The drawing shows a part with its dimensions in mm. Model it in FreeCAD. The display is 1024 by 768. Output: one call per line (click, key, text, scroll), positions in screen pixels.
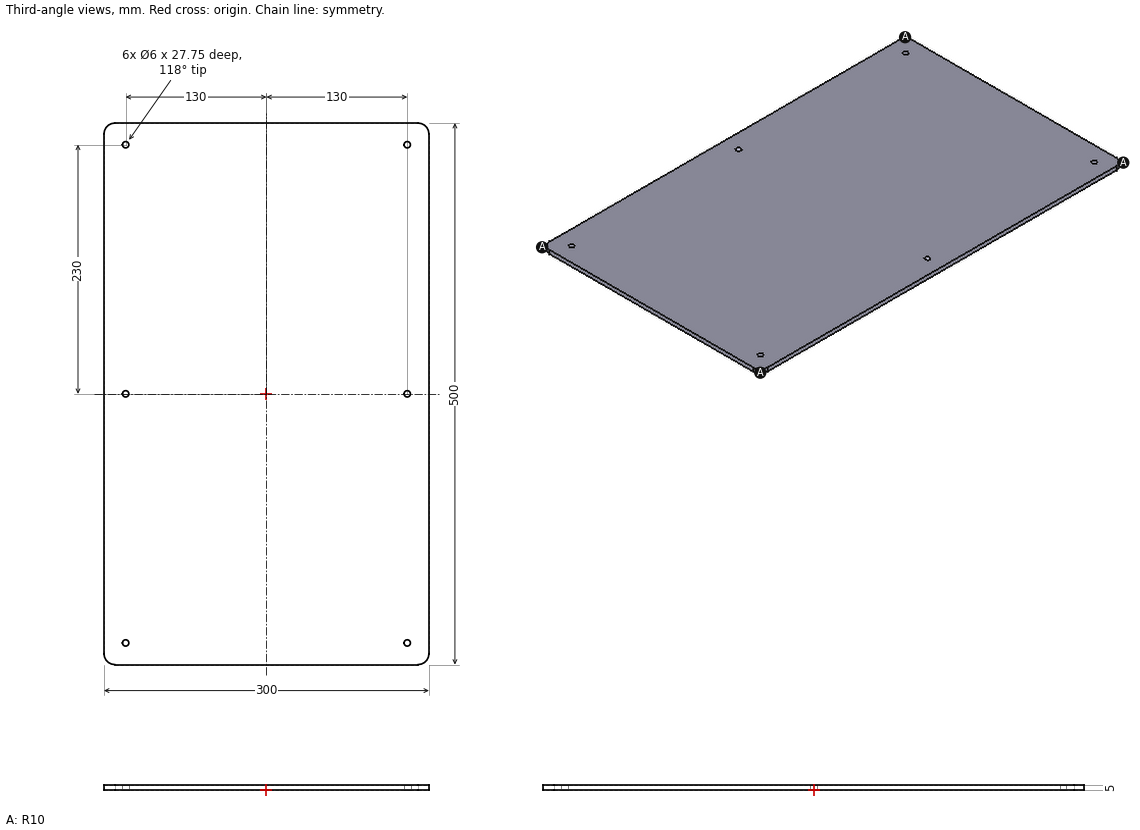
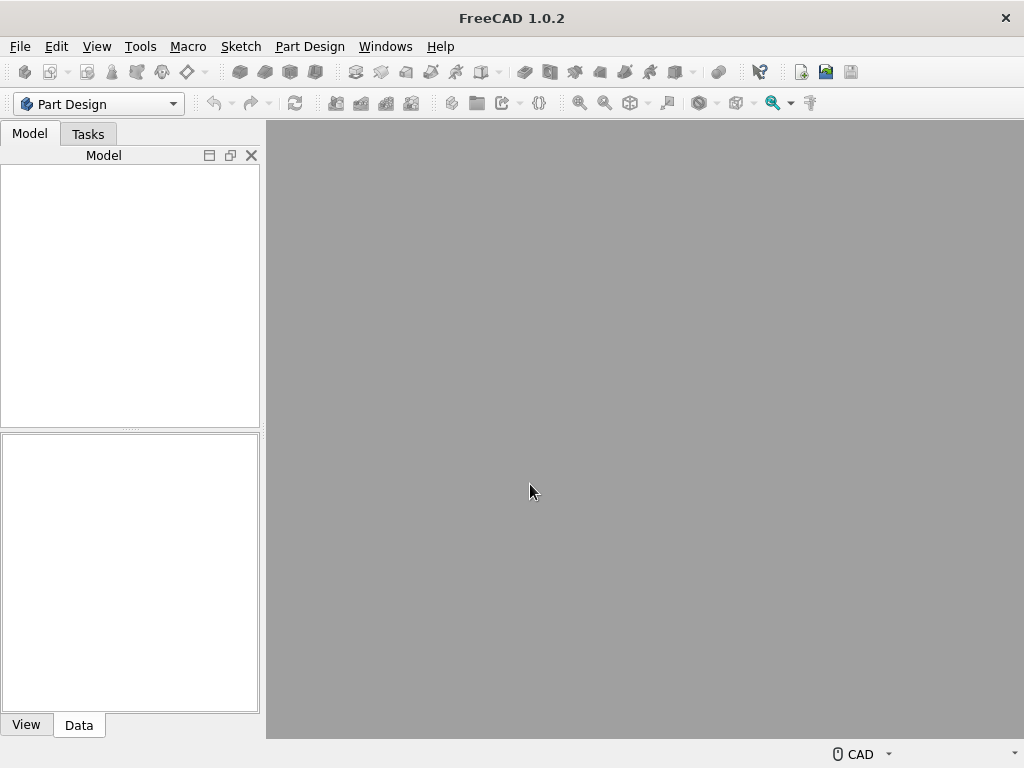
click(801, 72)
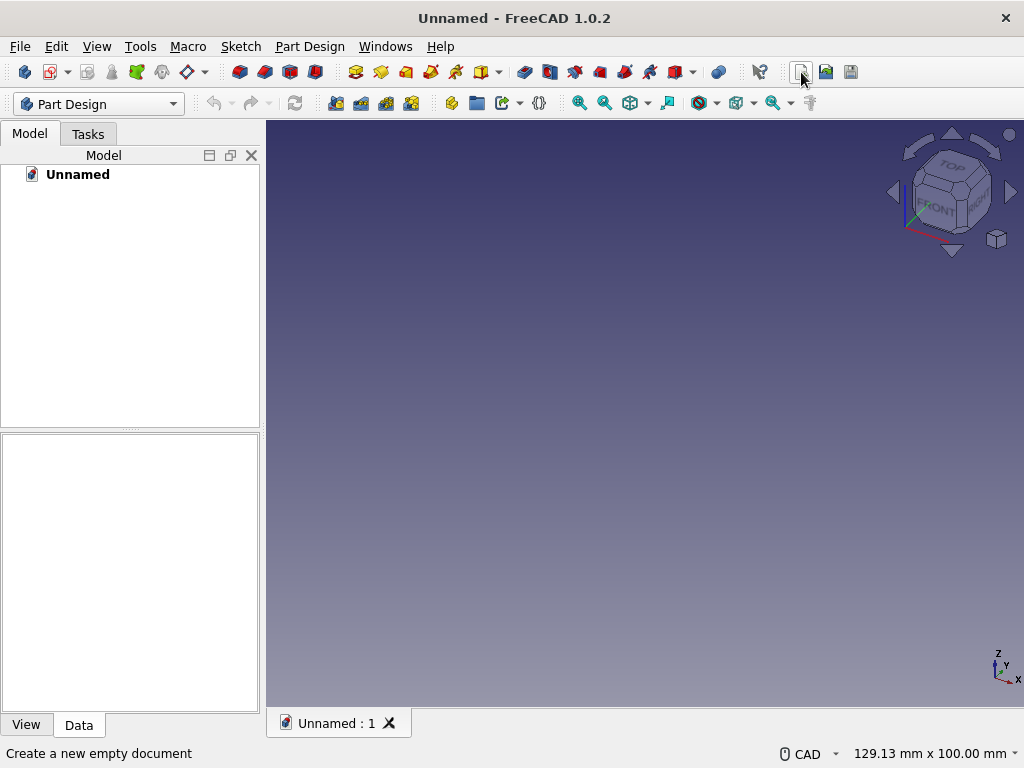
click(50, 72)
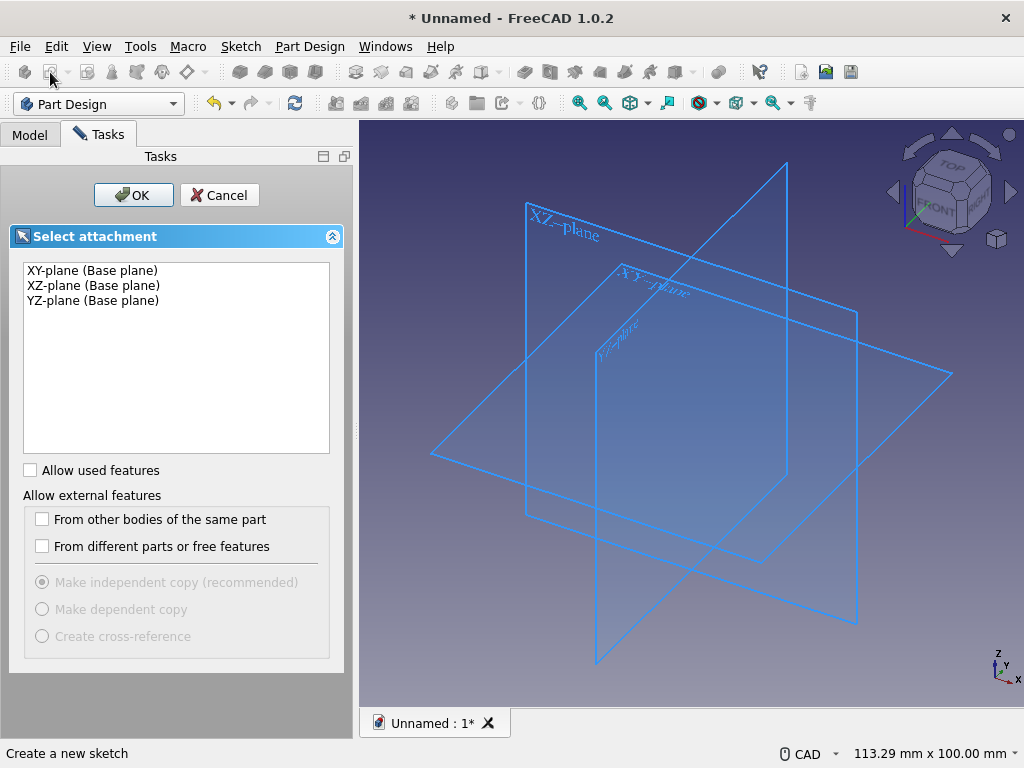
click(84, 270)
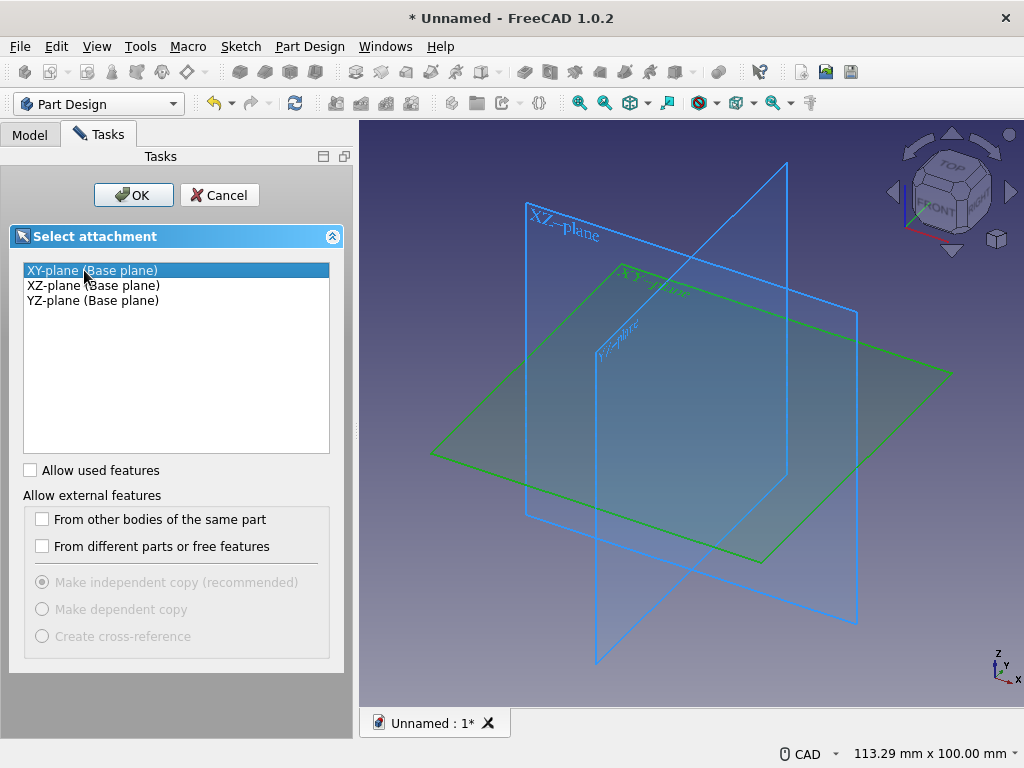
click(134, 195)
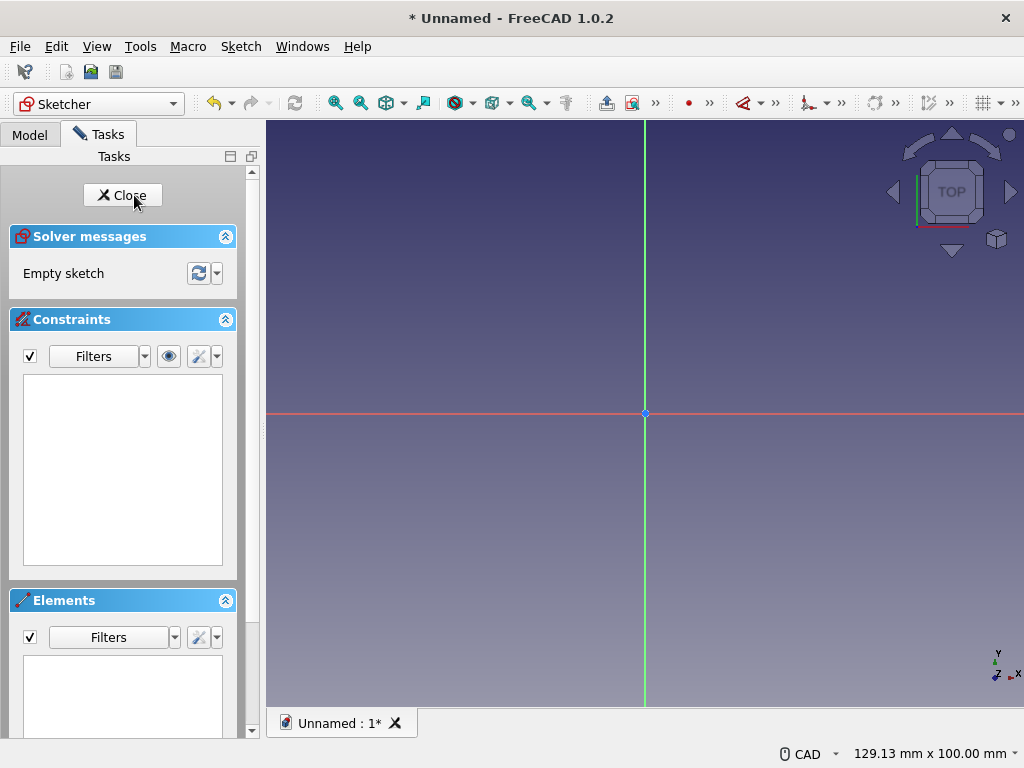
scroll(566, 414, down, 10)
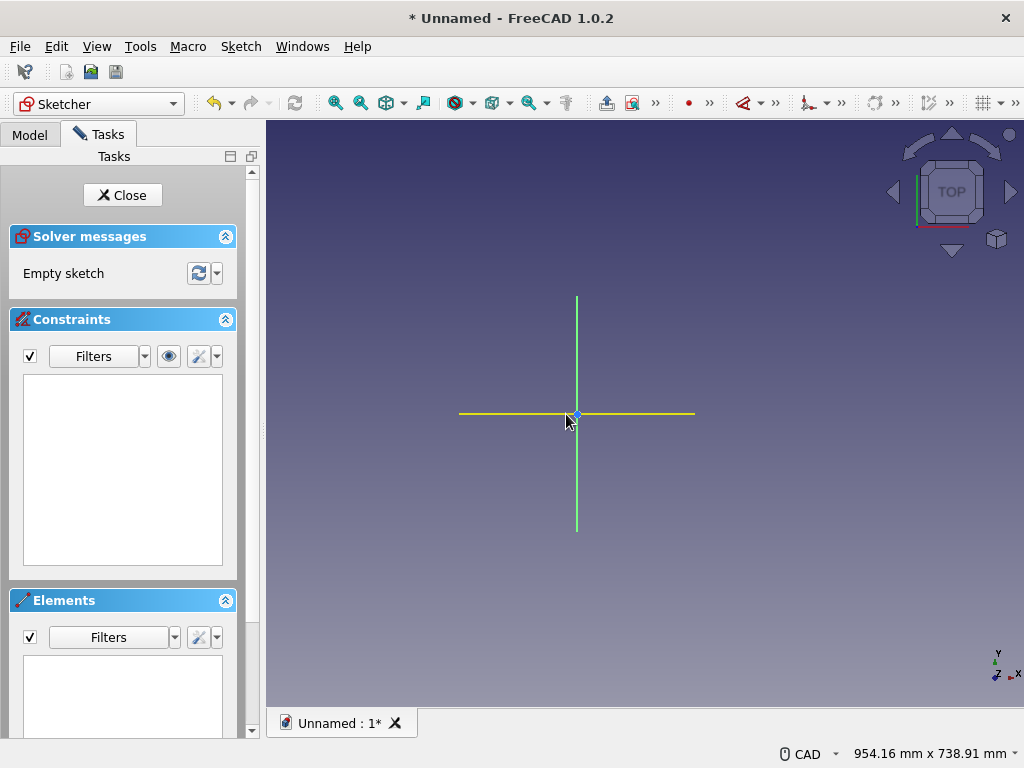
key(g)
key(v)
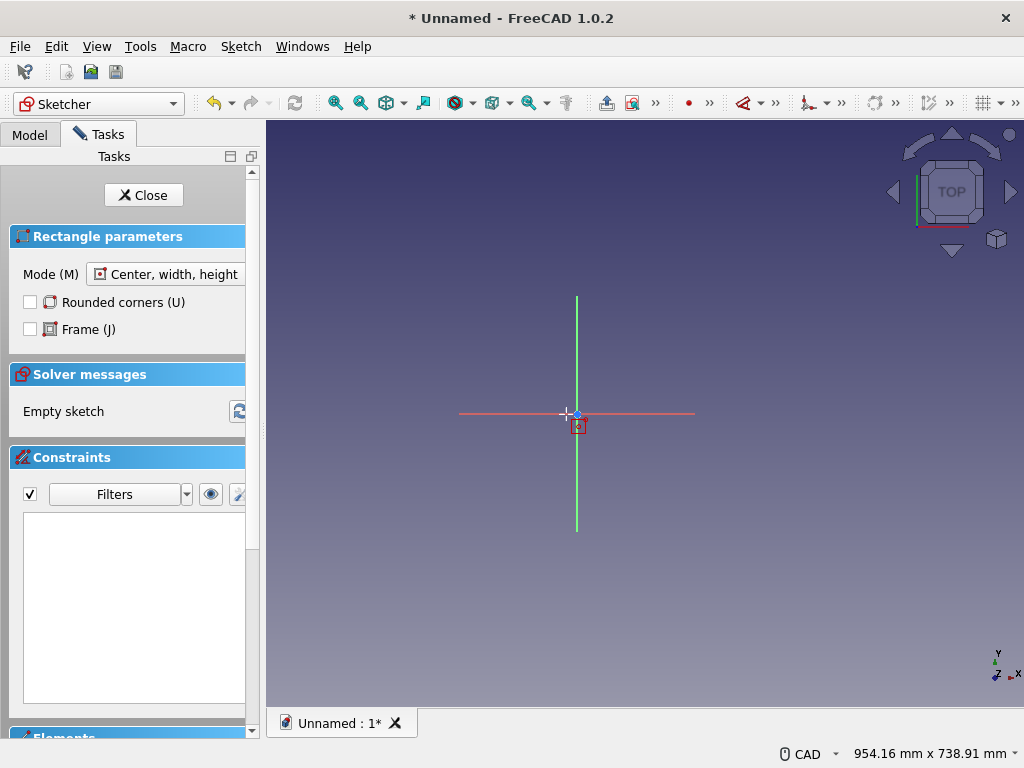
click(577, 414)
move(696, 216)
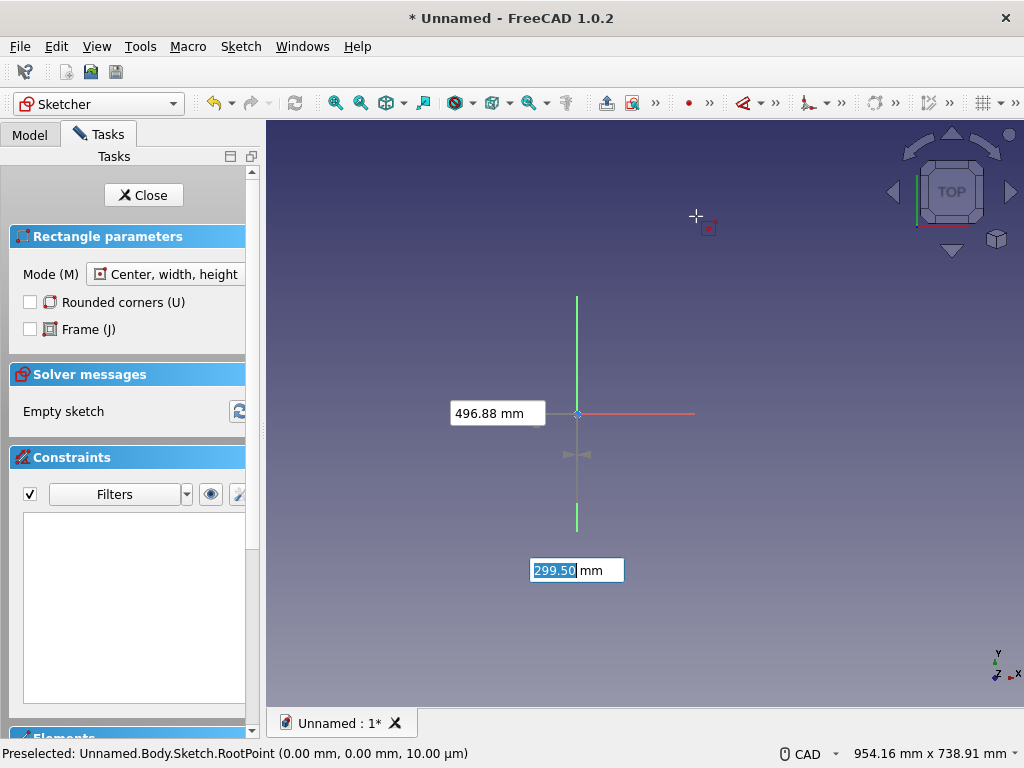
text(300)
key(Tab)
text(500)
key(Return)
key(Escape)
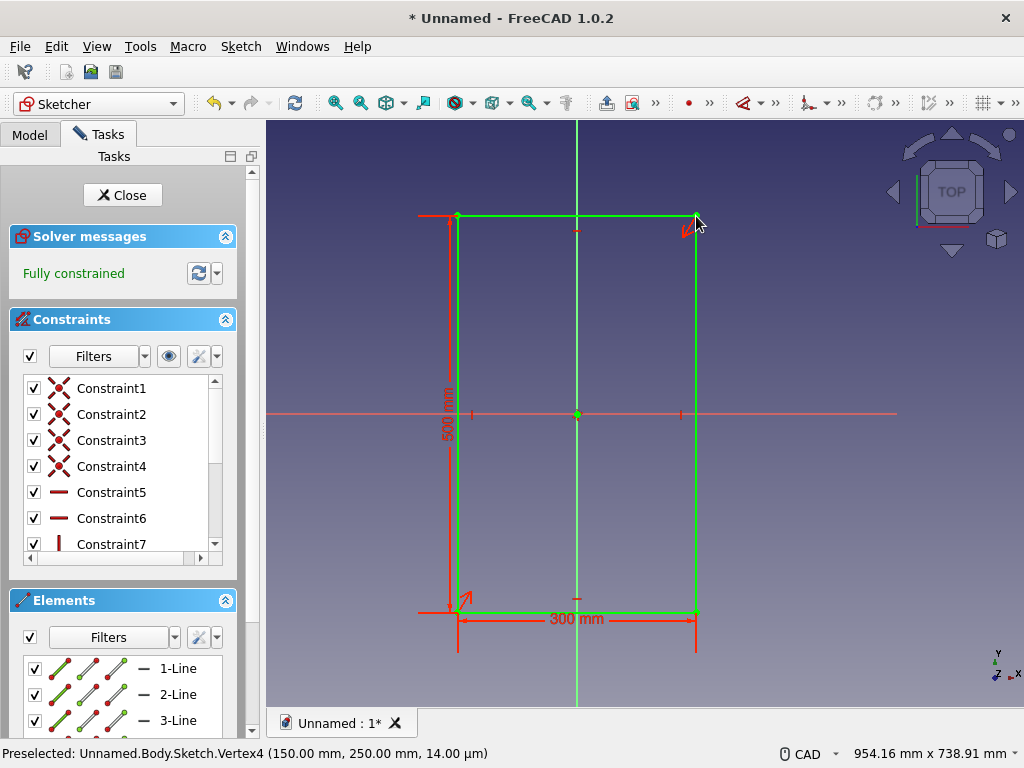
click(123, 195)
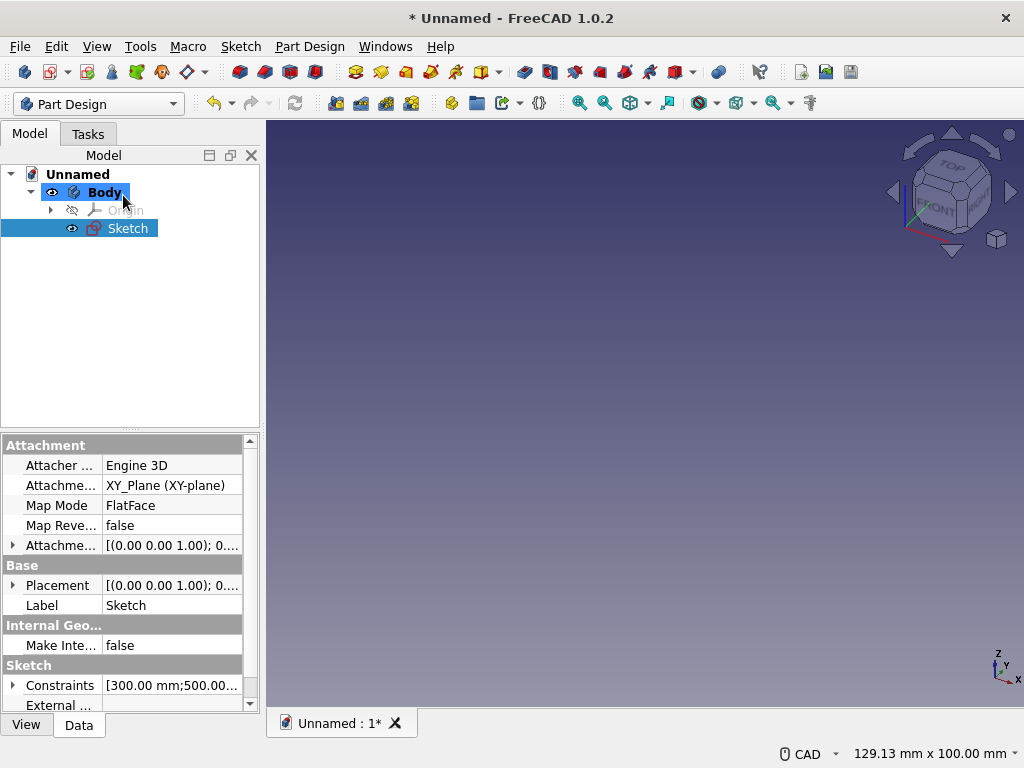
click(356, 72)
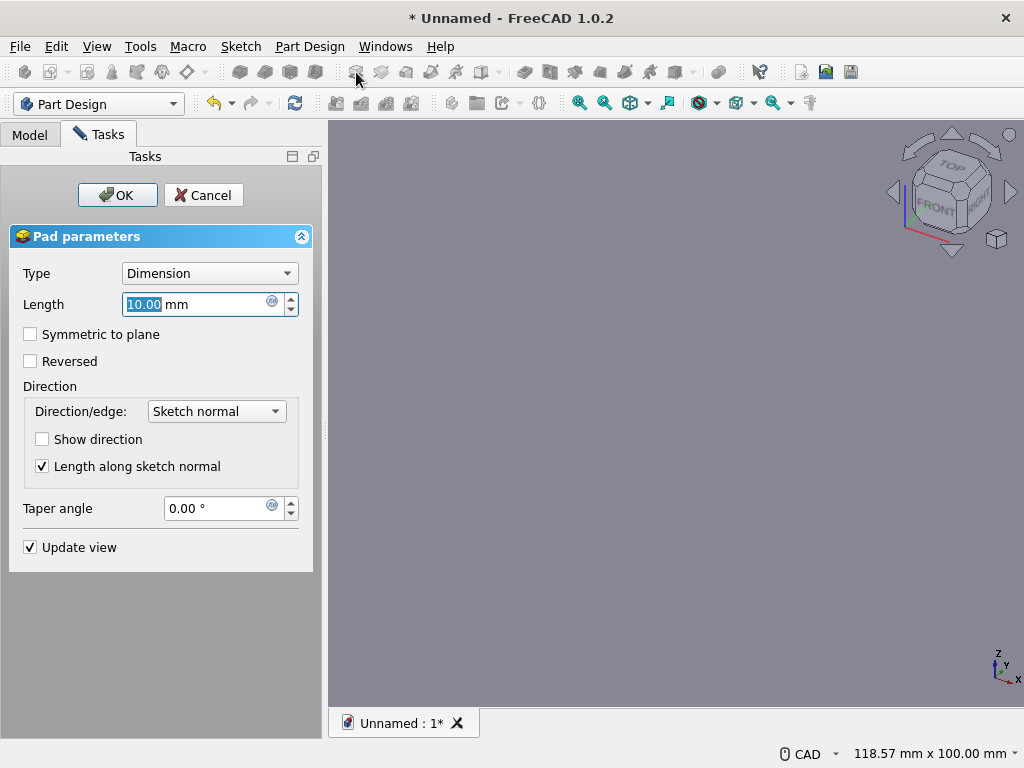
text(5)
key(Tab)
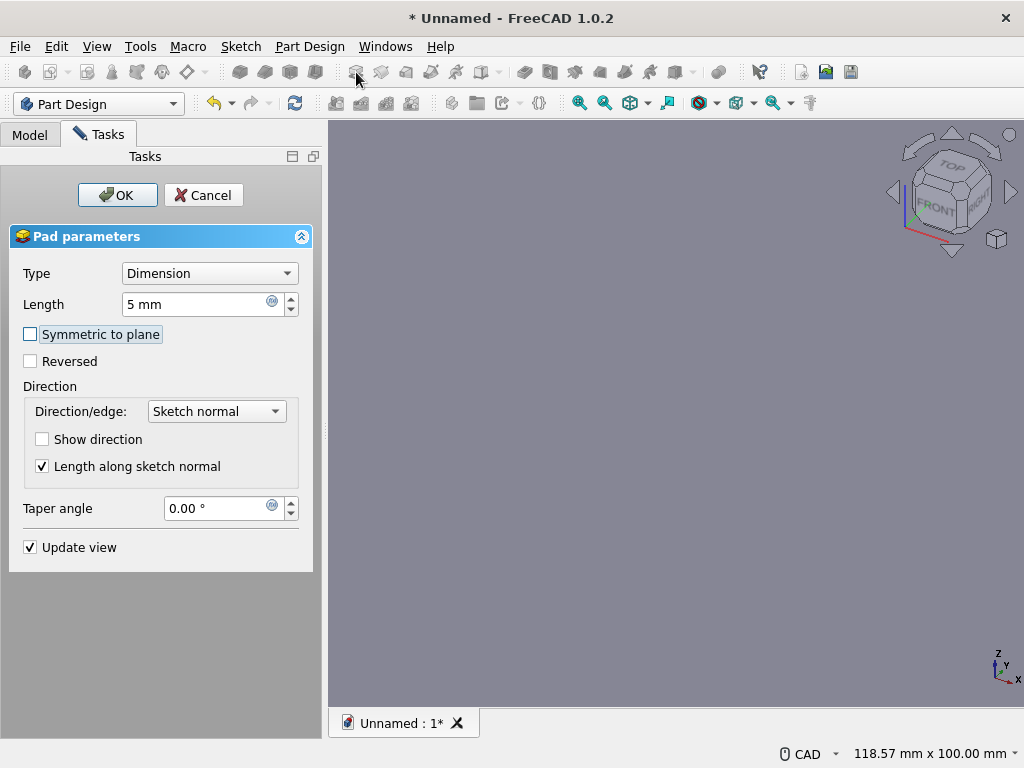
click(118, 195)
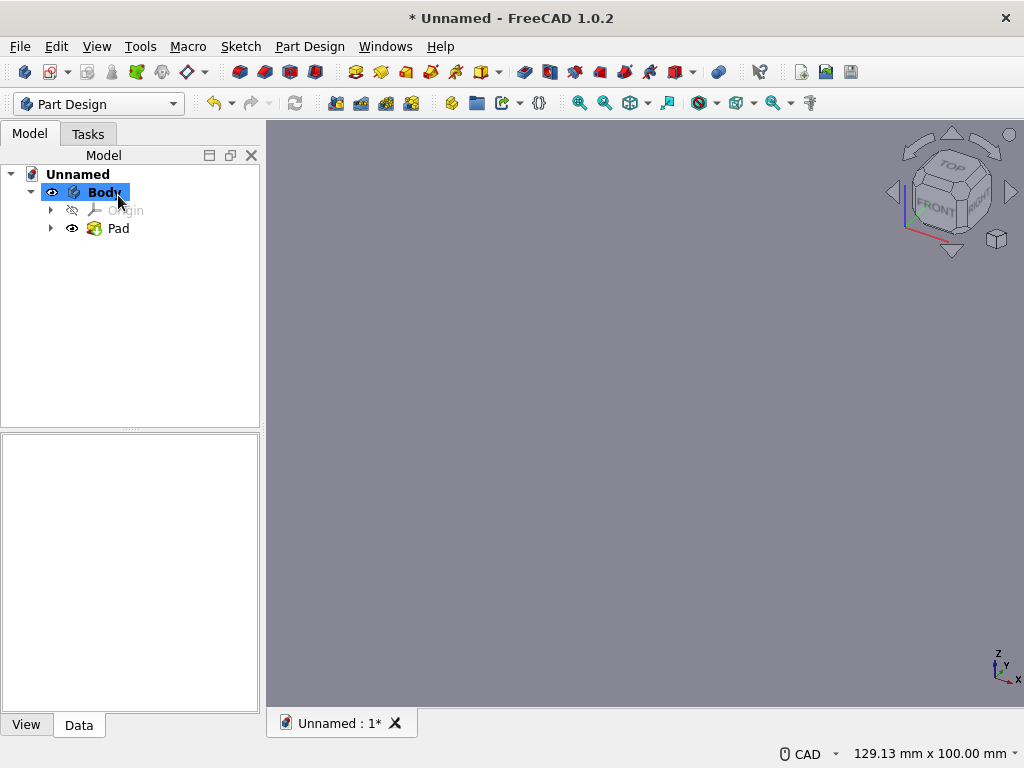
click(580, 104)